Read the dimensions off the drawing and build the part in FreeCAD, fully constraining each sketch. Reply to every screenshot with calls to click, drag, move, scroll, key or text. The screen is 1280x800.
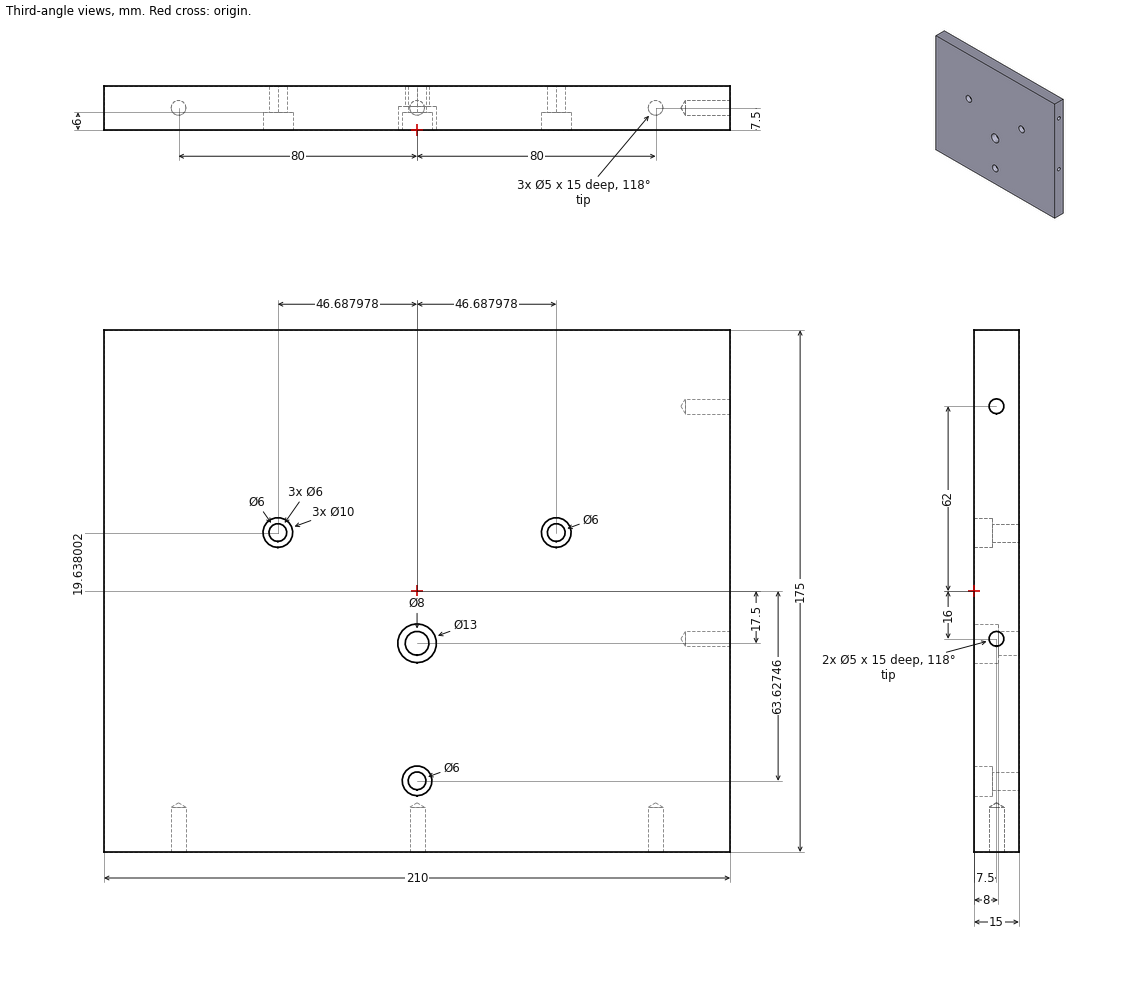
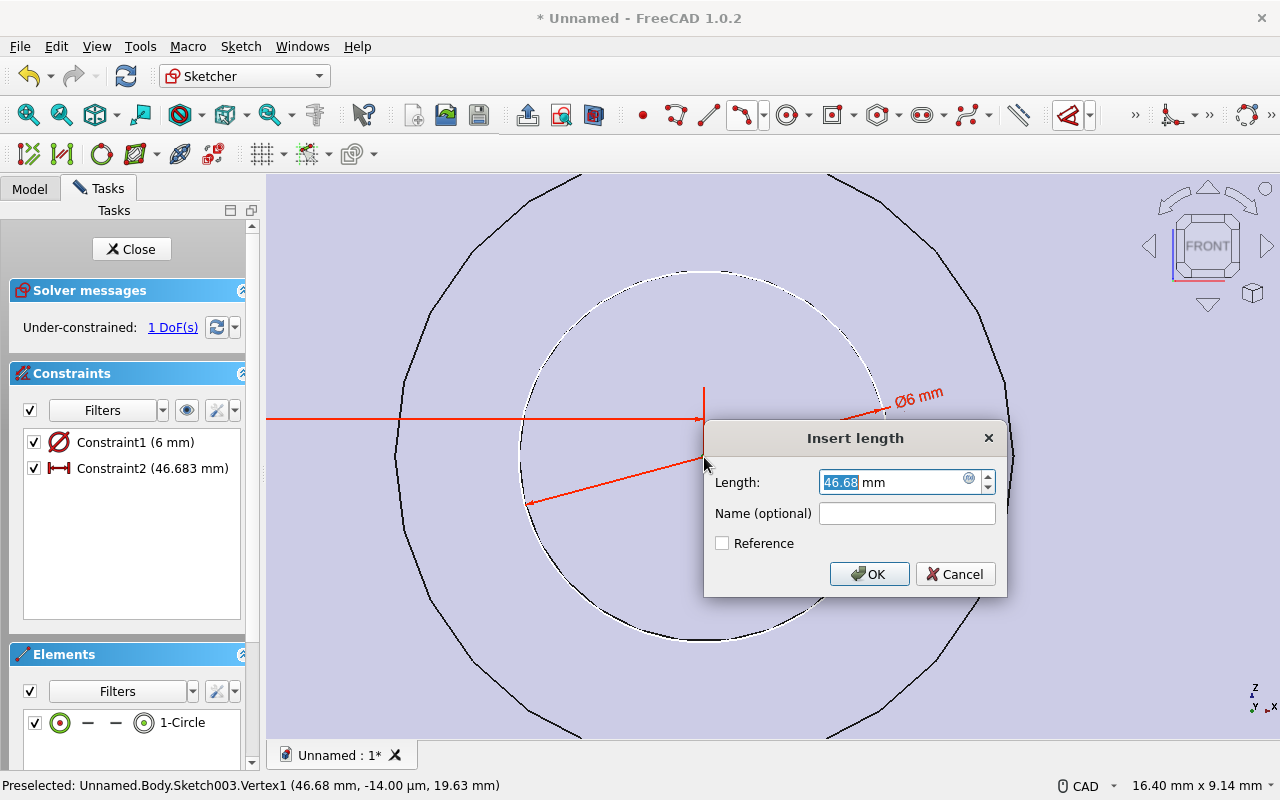
text(46.687978)
key(Return)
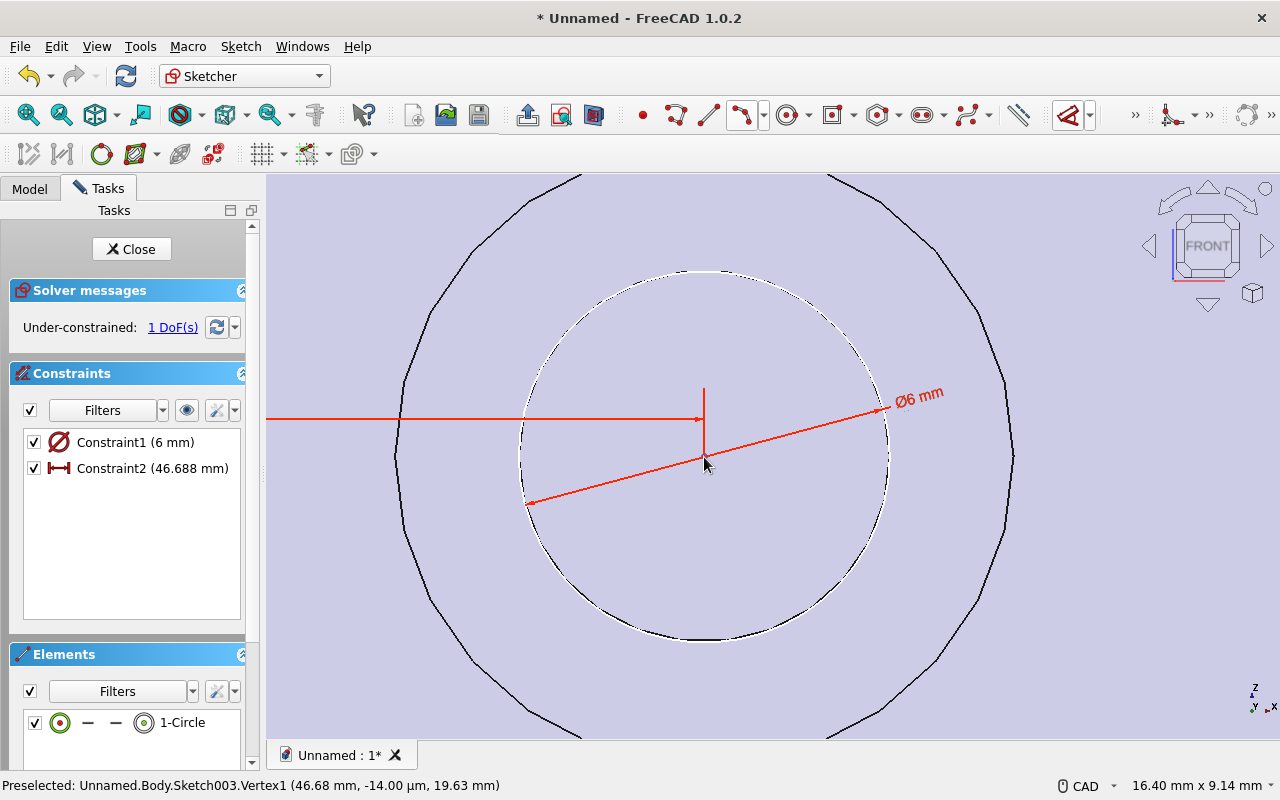
click(704, 457)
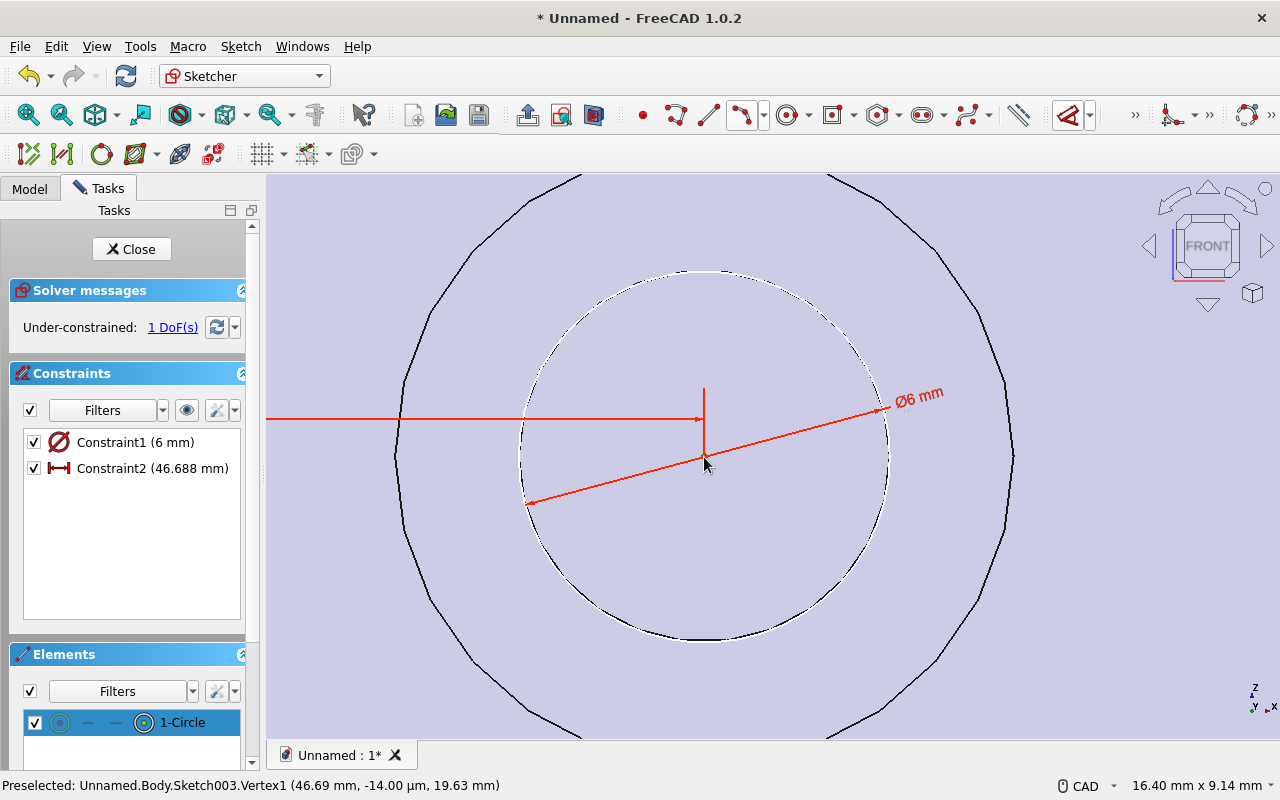
key(i)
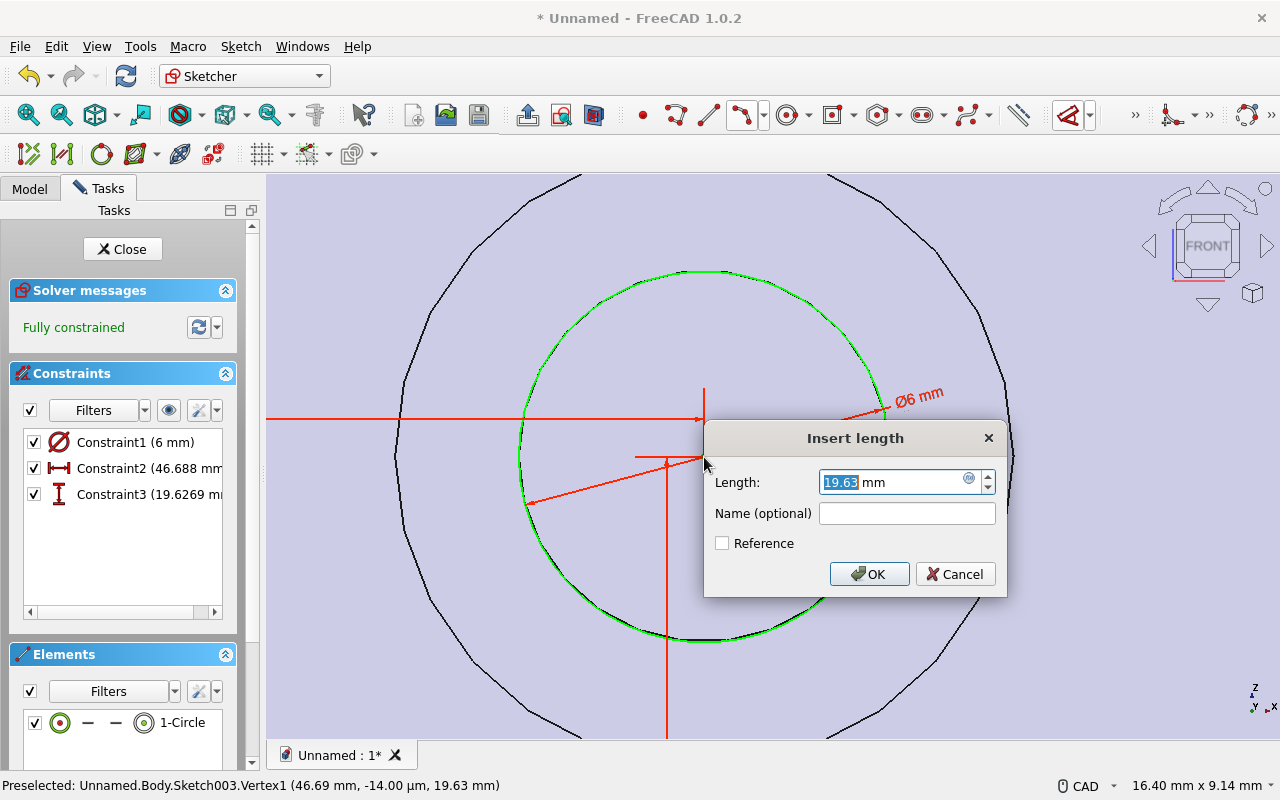
text(19.638002)
key(Return)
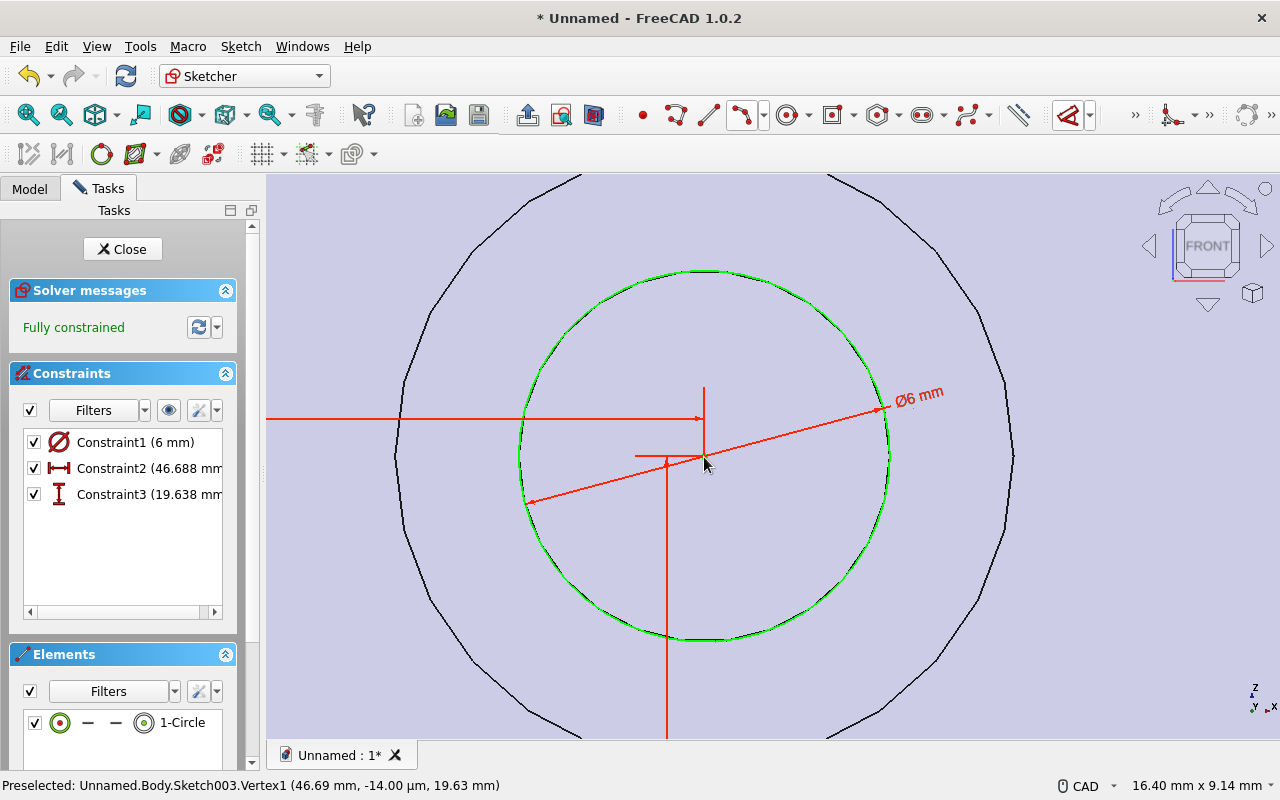
click(123, 249)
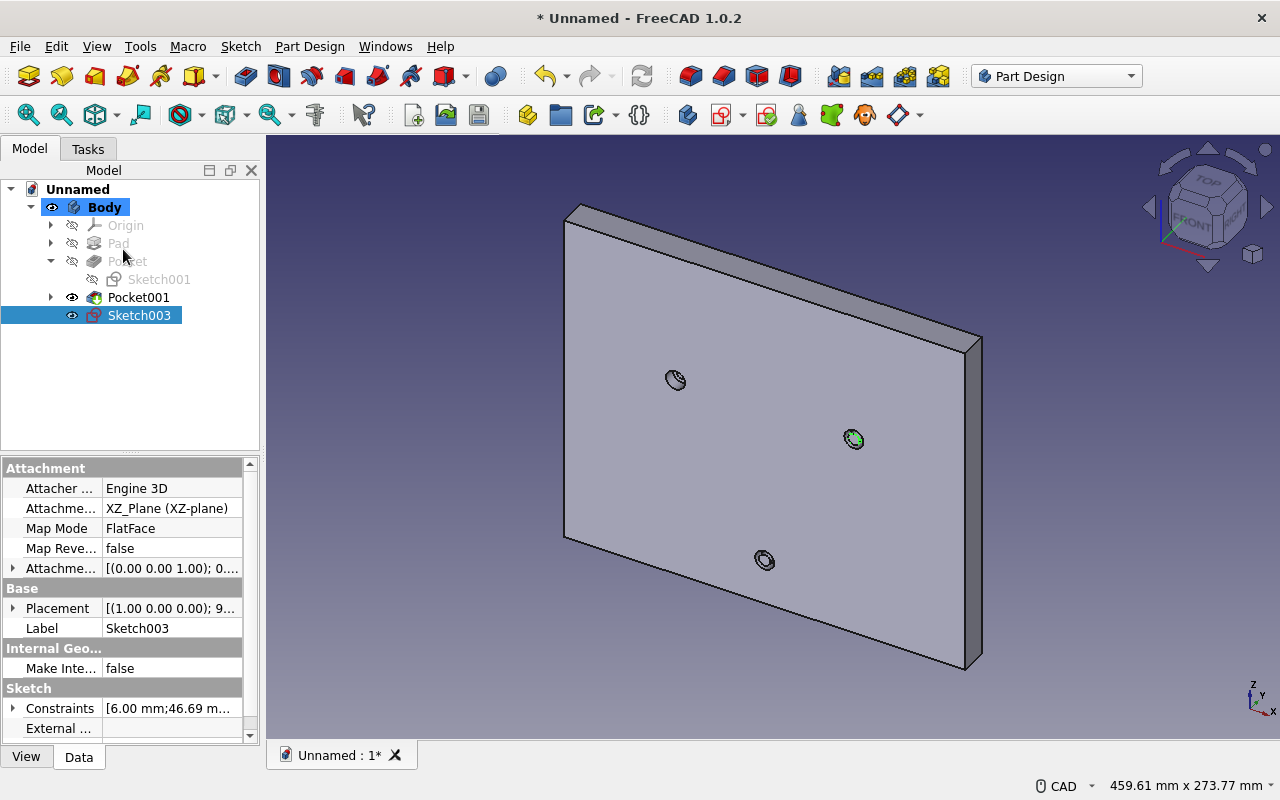
click(246, 76)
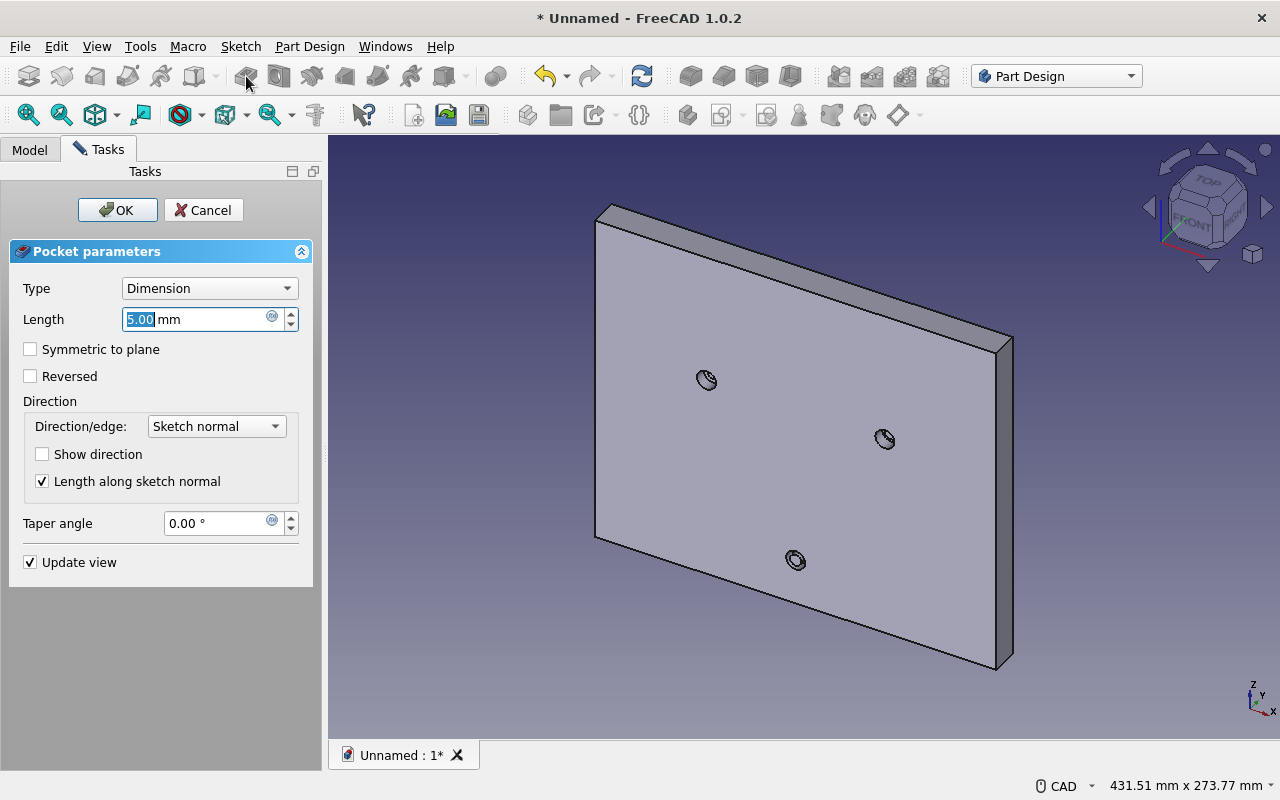
click(210, 288)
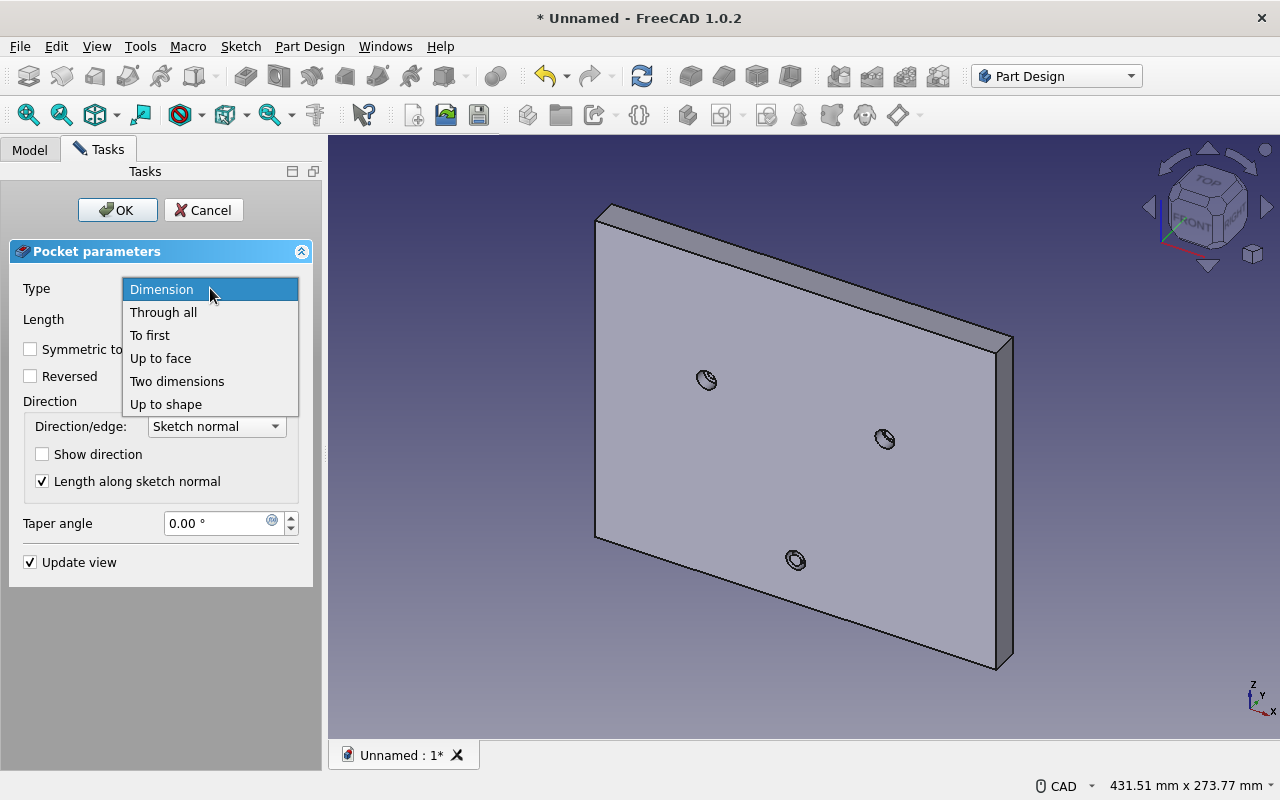
click(208, 336)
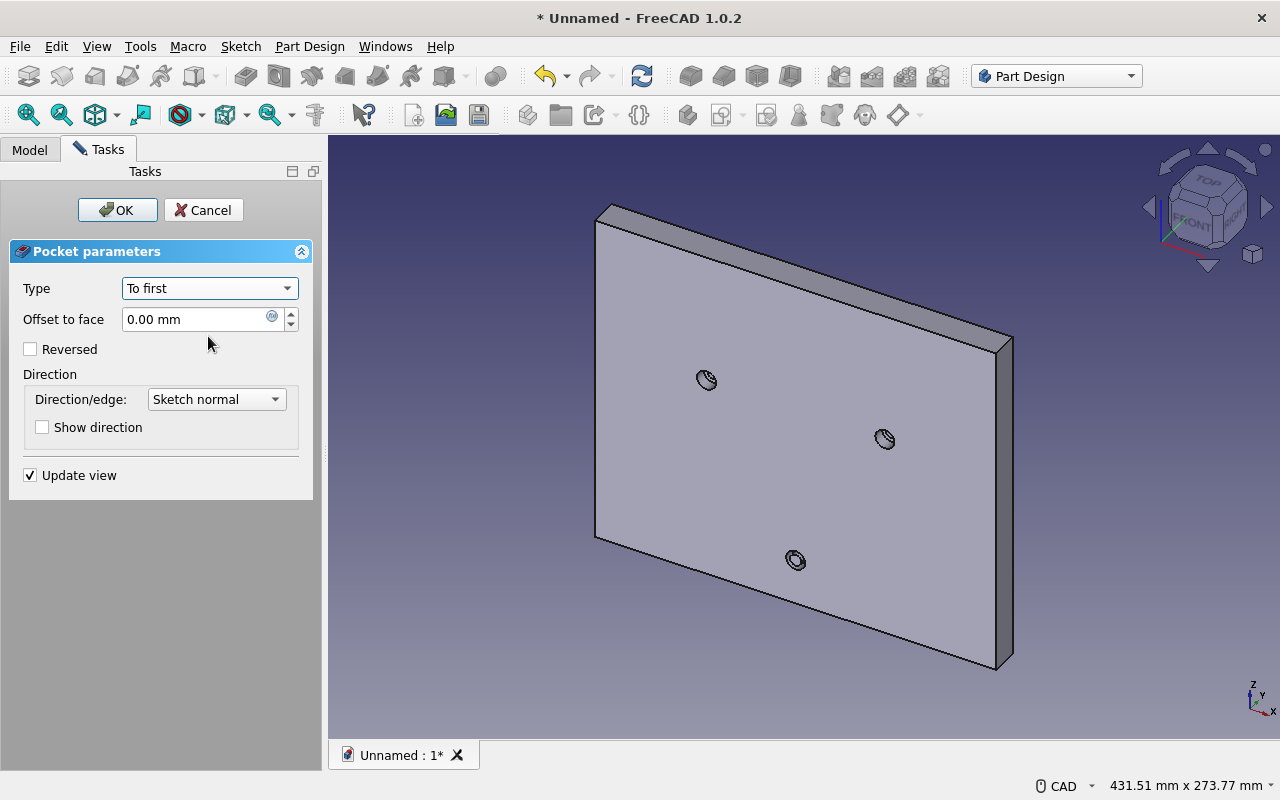
click(118, 210)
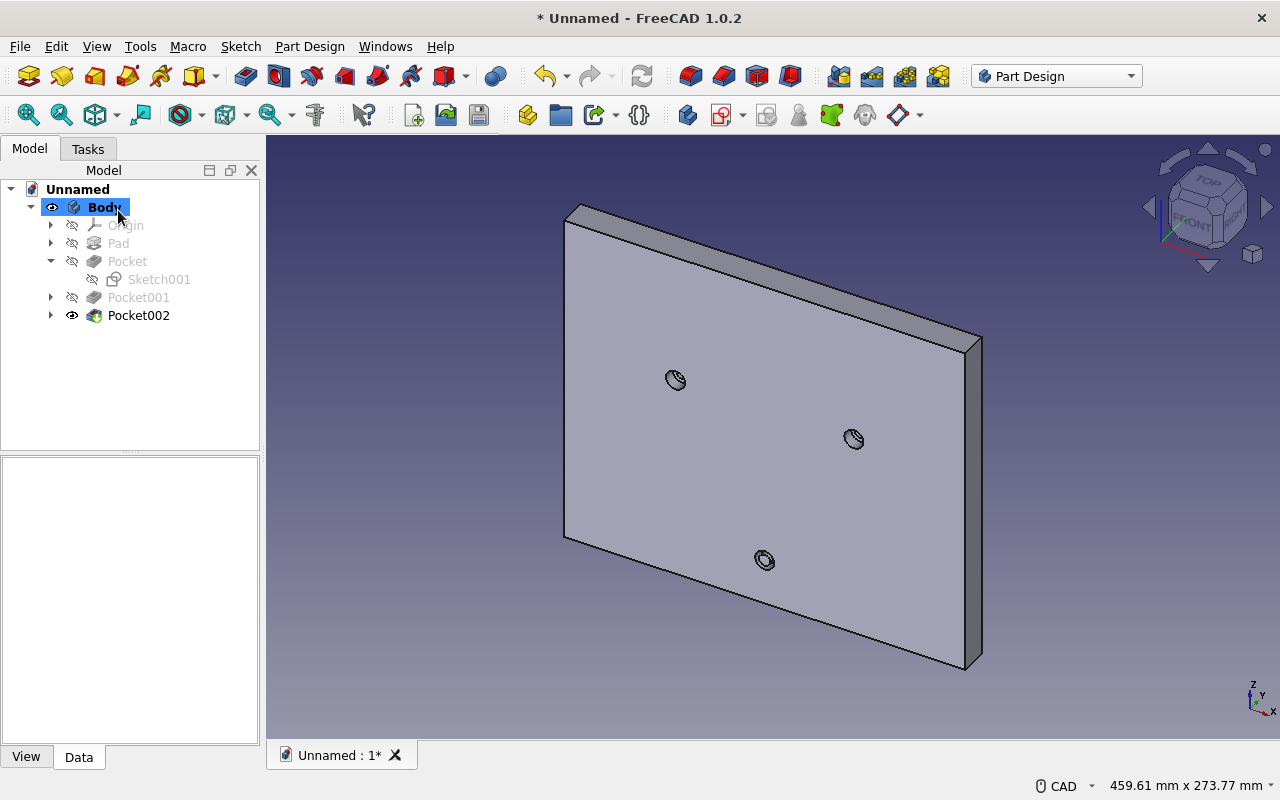
click(765, 444)